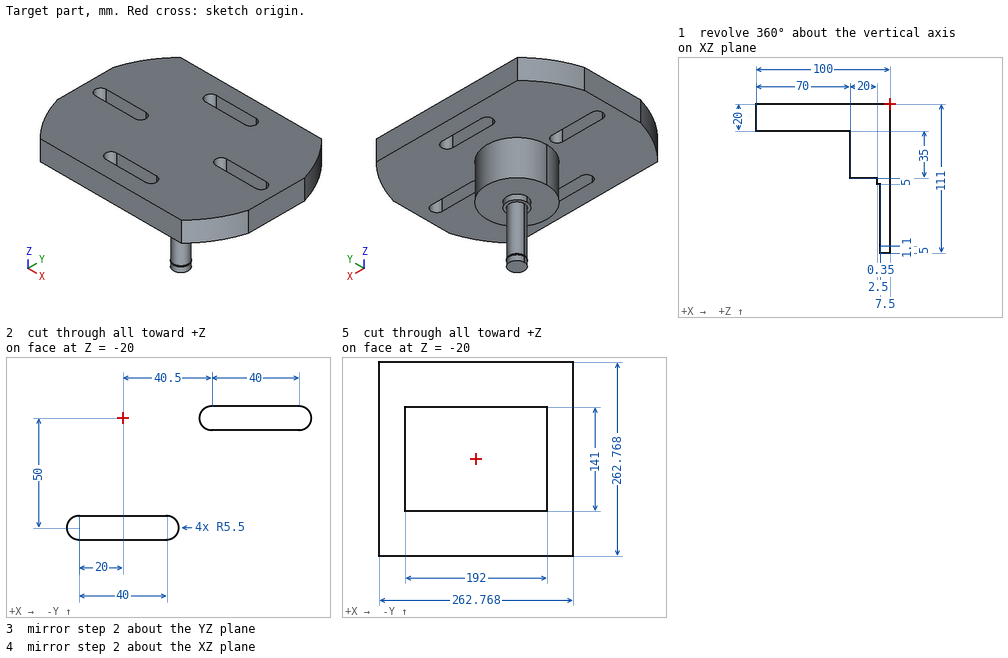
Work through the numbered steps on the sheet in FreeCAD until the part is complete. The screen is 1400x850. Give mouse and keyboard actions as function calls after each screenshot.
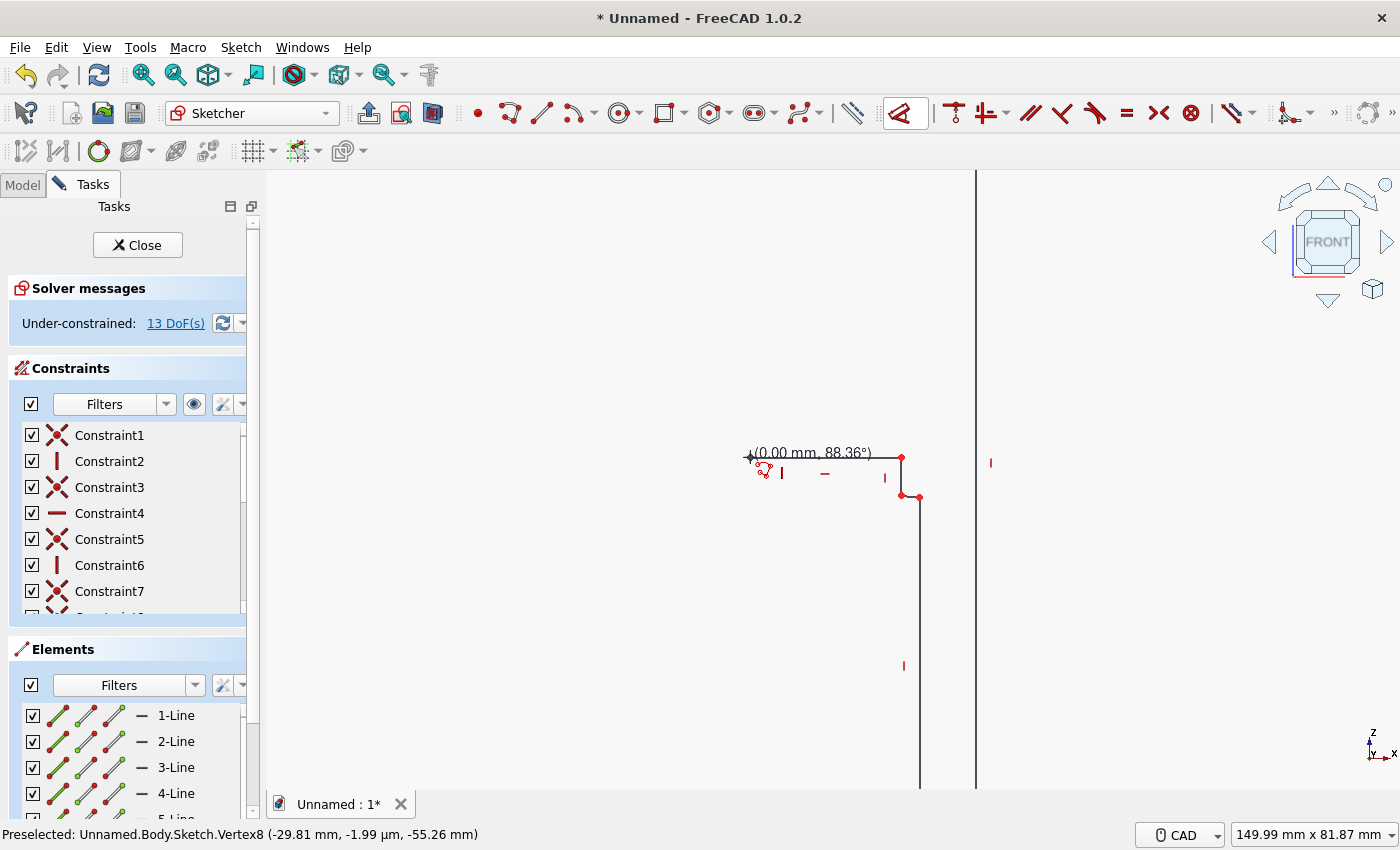
scroll(900, 495, down, 4)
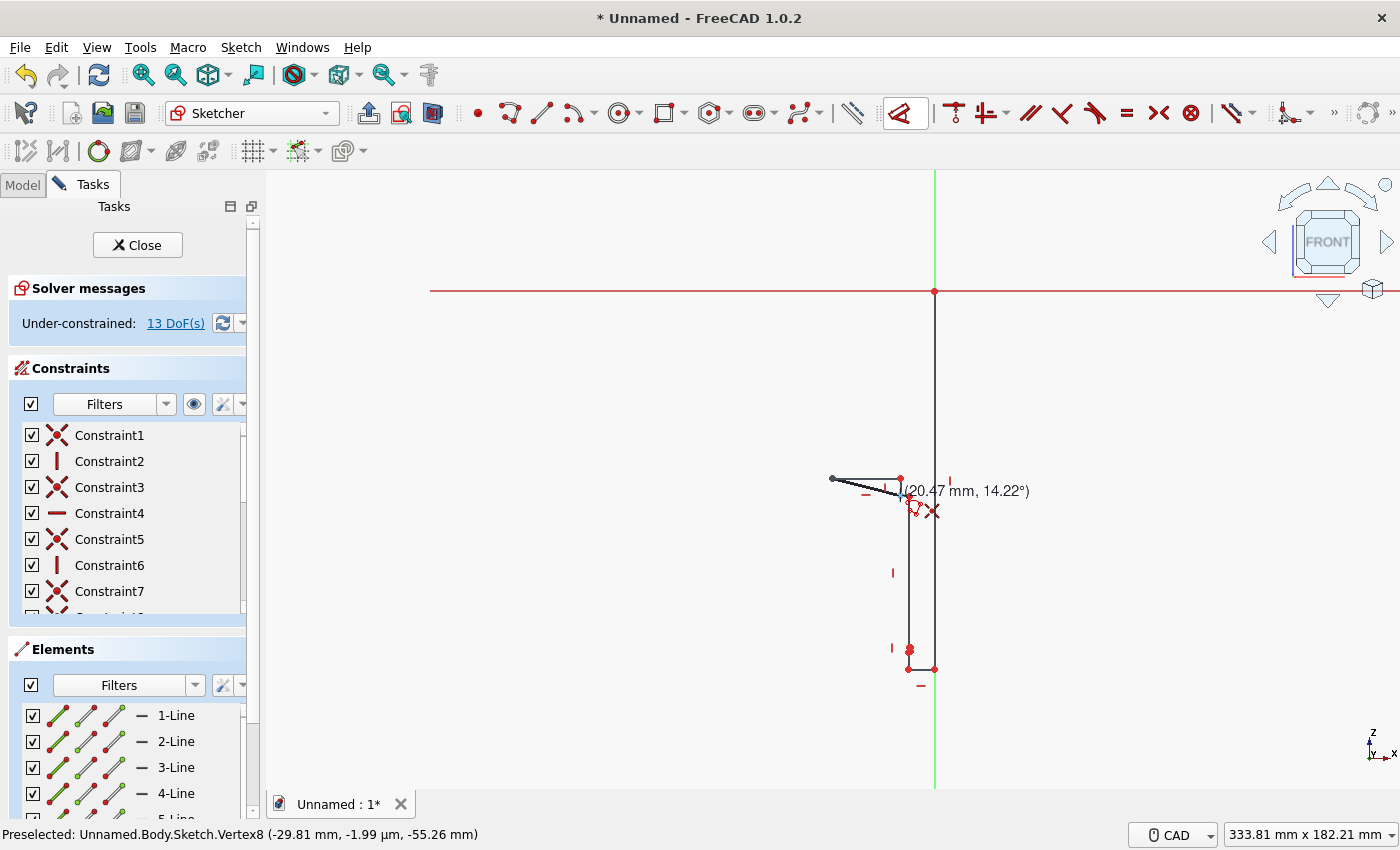
click(833, 359)
click(595, 359)
click(595, 300)
click(935, 291)
key(Escape)
key(Escape)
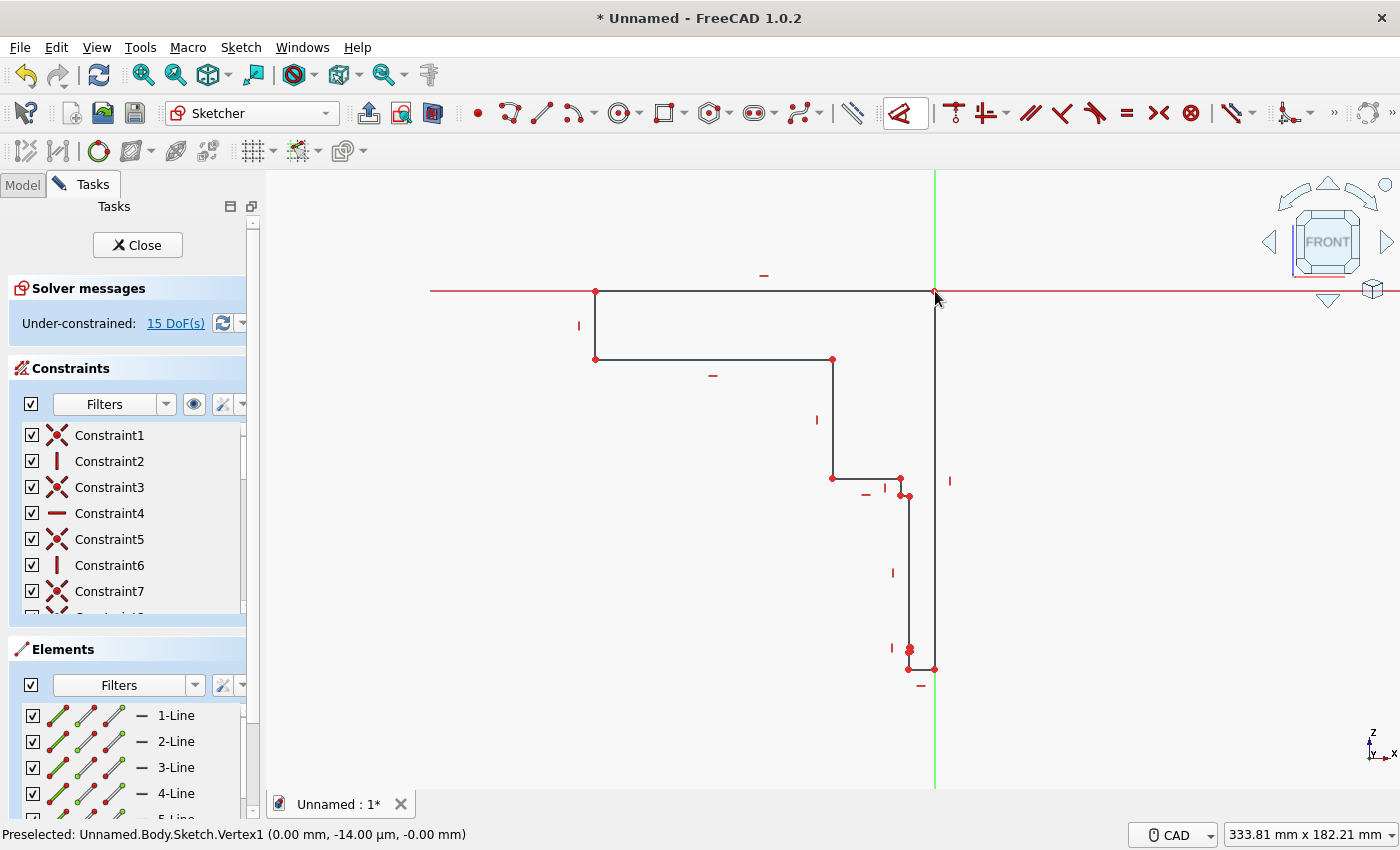
scroll(910, 652, up, 14)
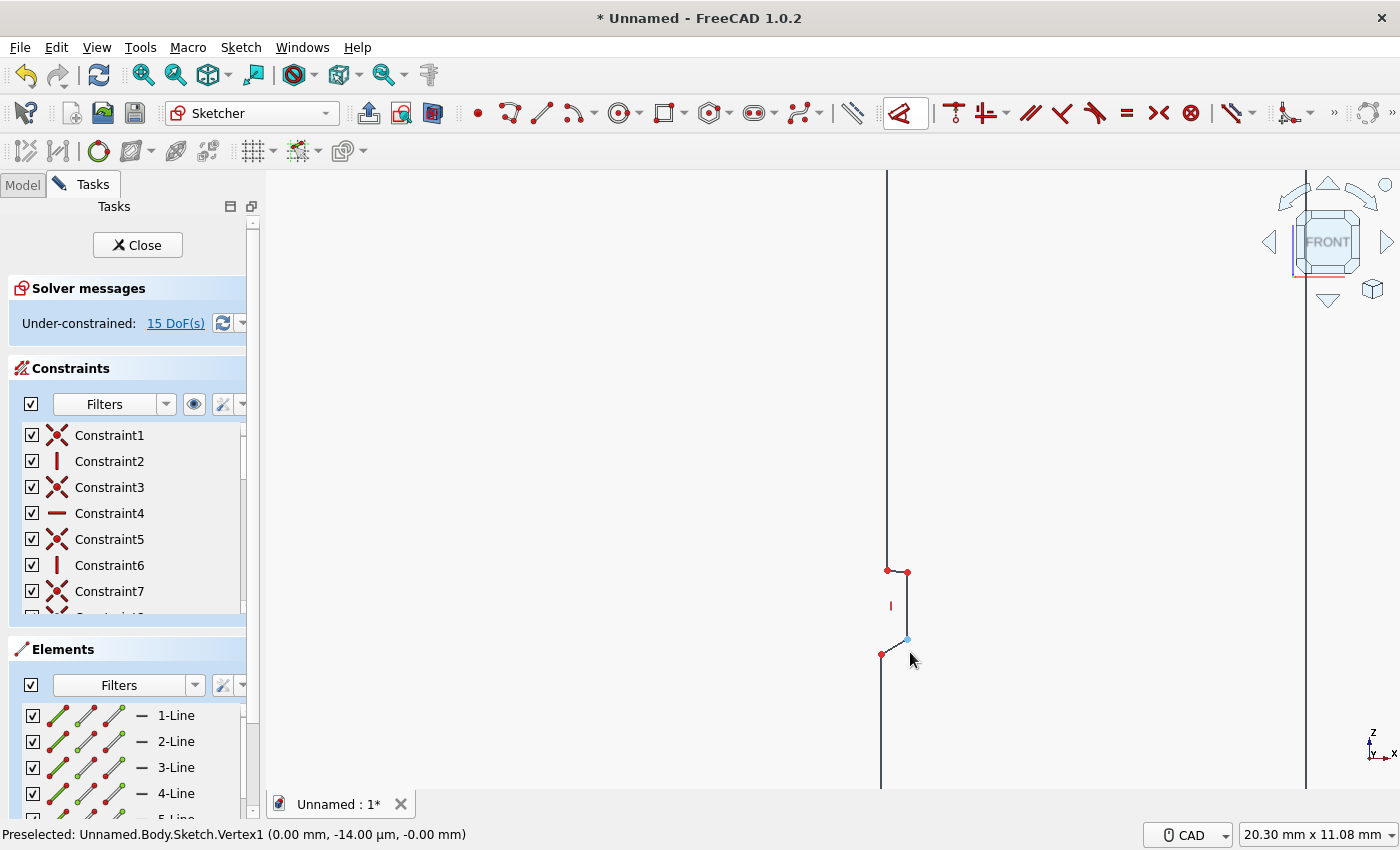
click(894, 647)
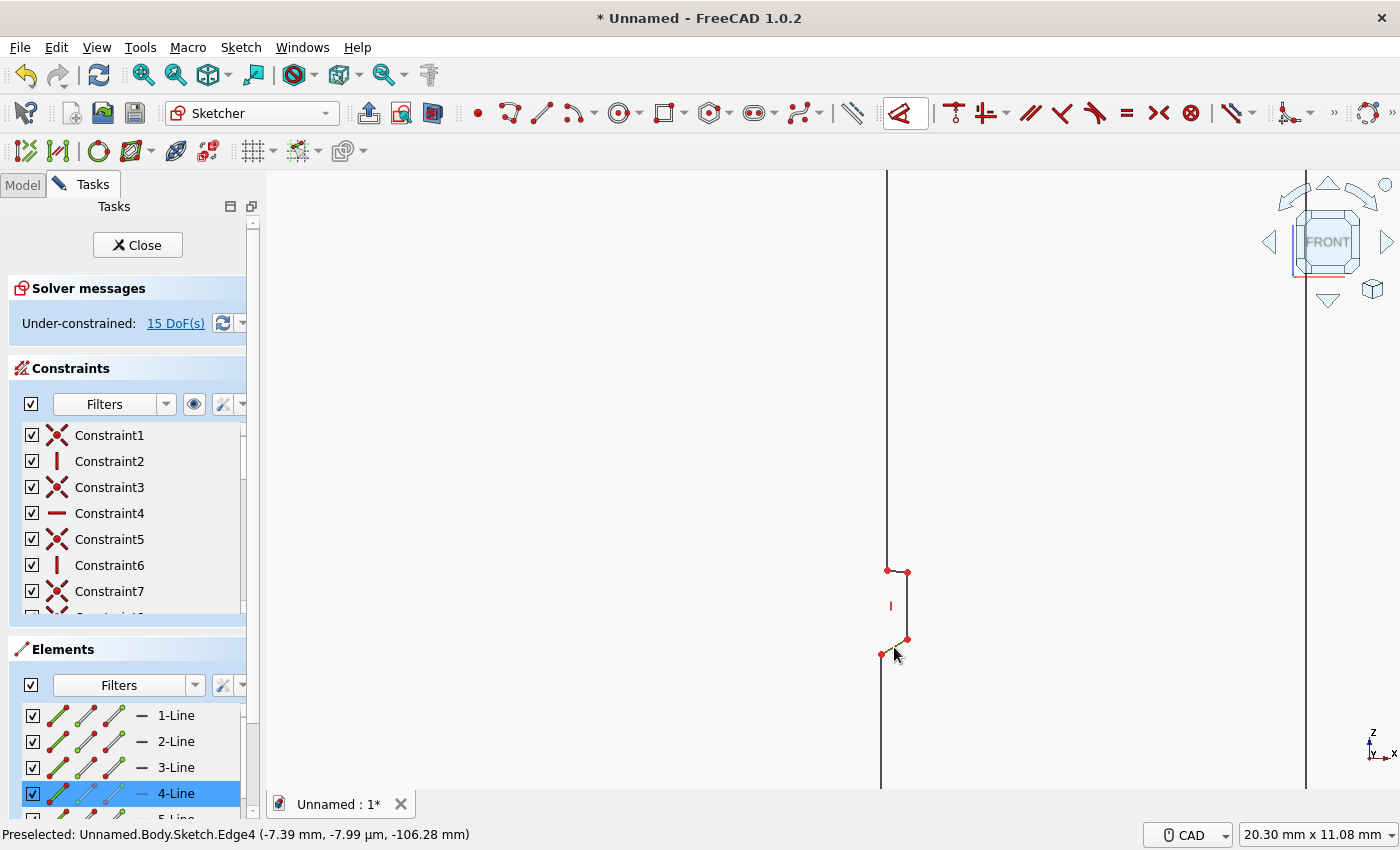
key(h)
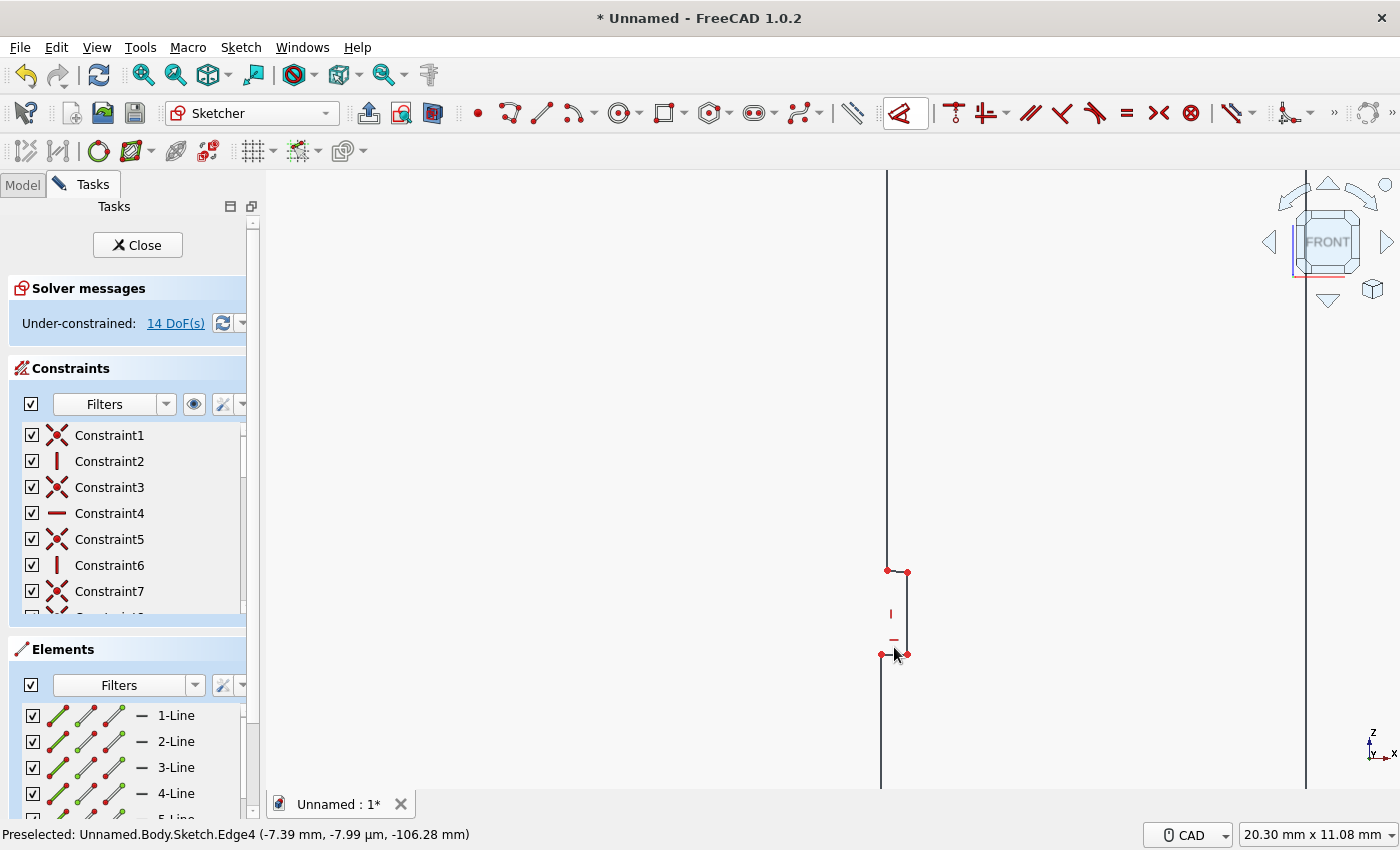
click(897, 572)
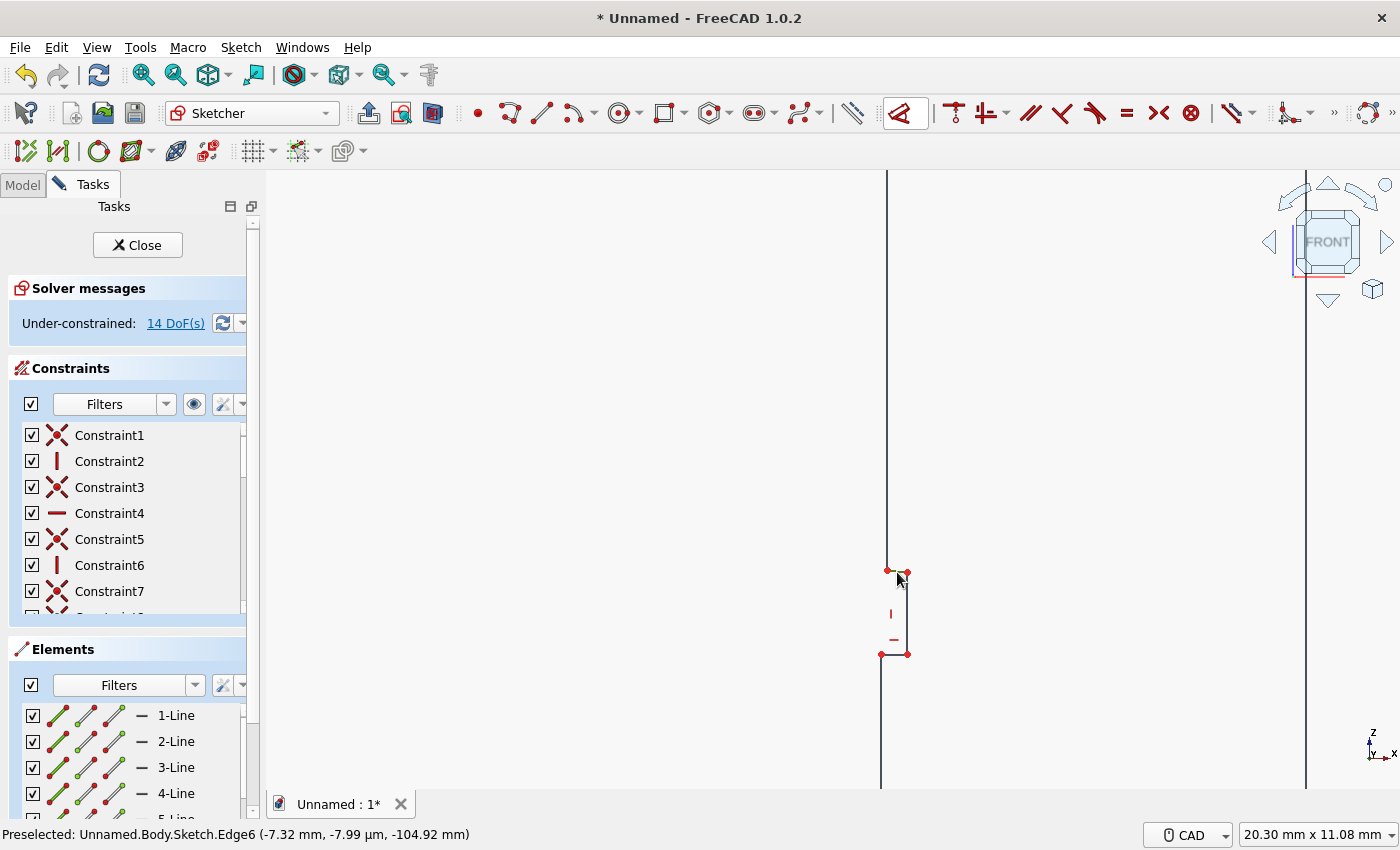
key(h)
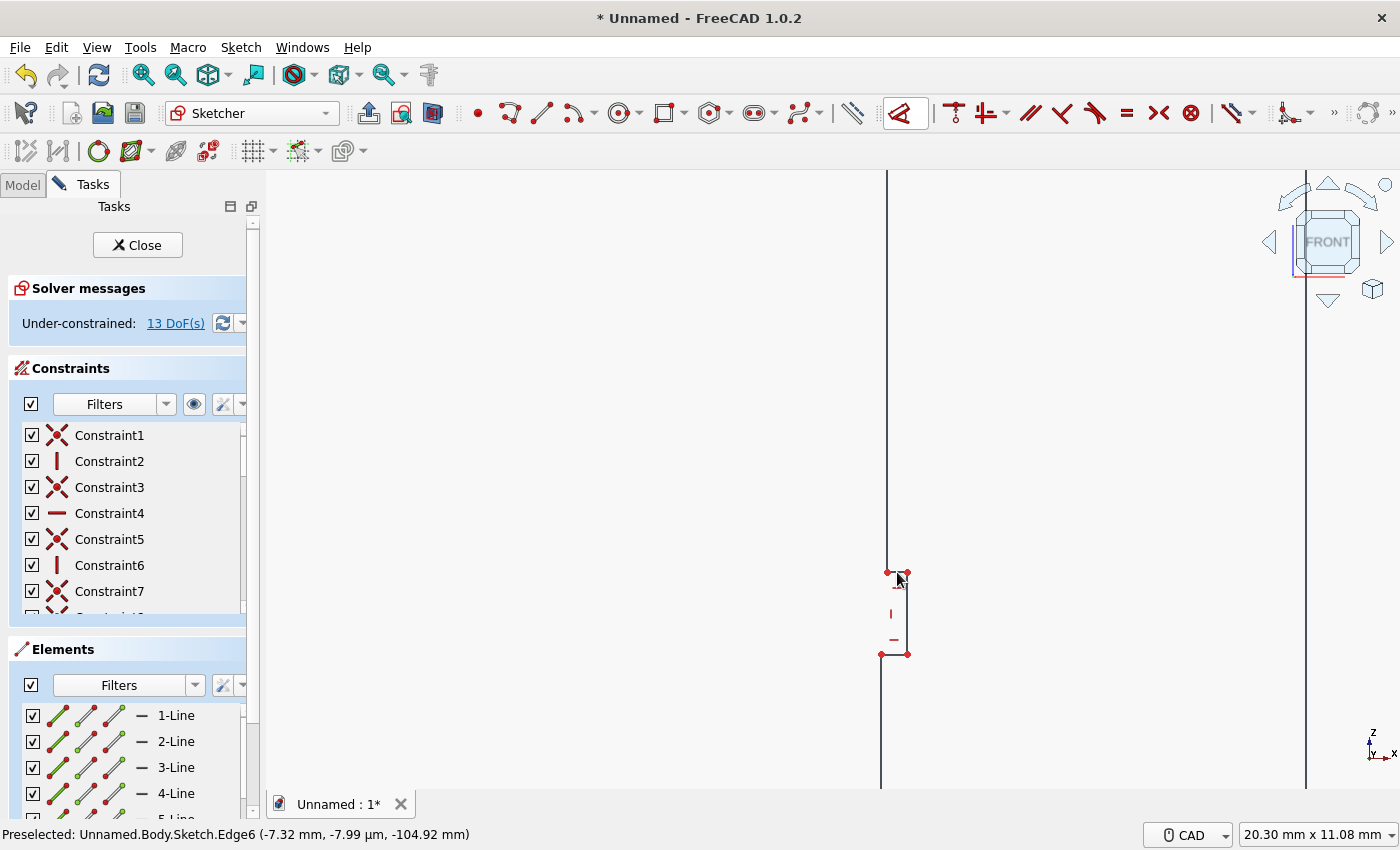
scroll(910, 652, down, 14)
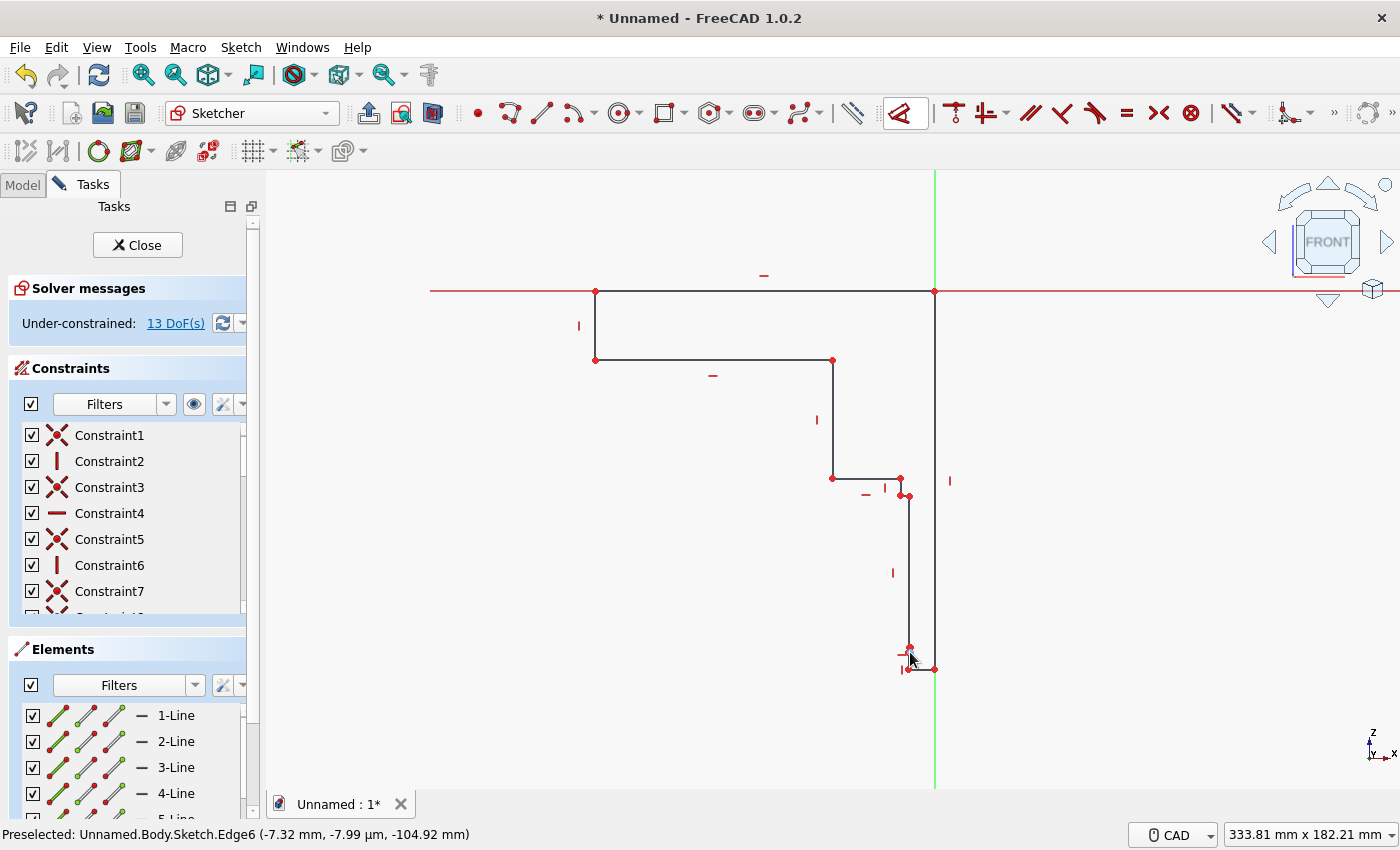
scroll(907, 496, up, 9)